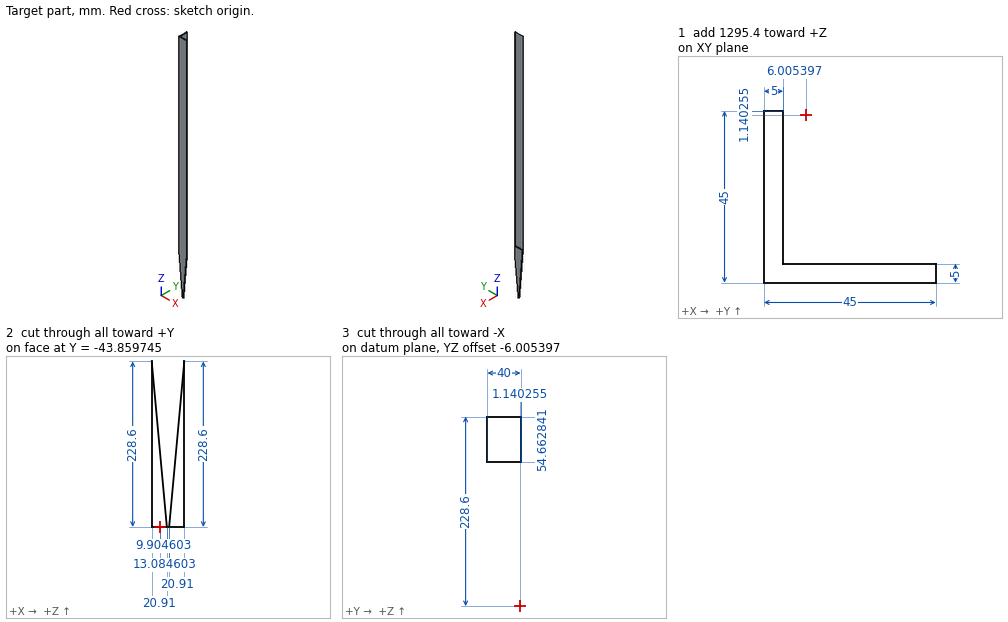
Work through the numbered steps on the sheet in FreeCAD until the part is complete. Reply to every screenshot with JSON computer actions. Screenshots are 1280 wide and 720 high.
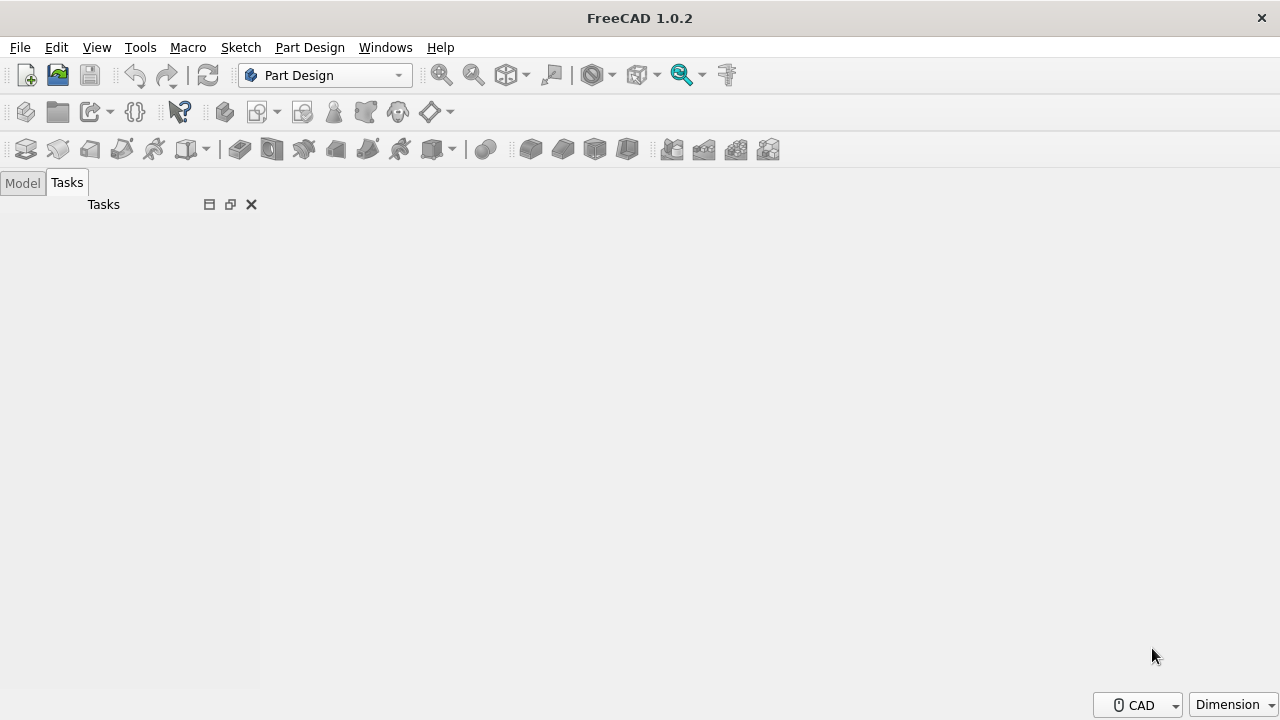
{"action": "key", "text": "ctrl+n"}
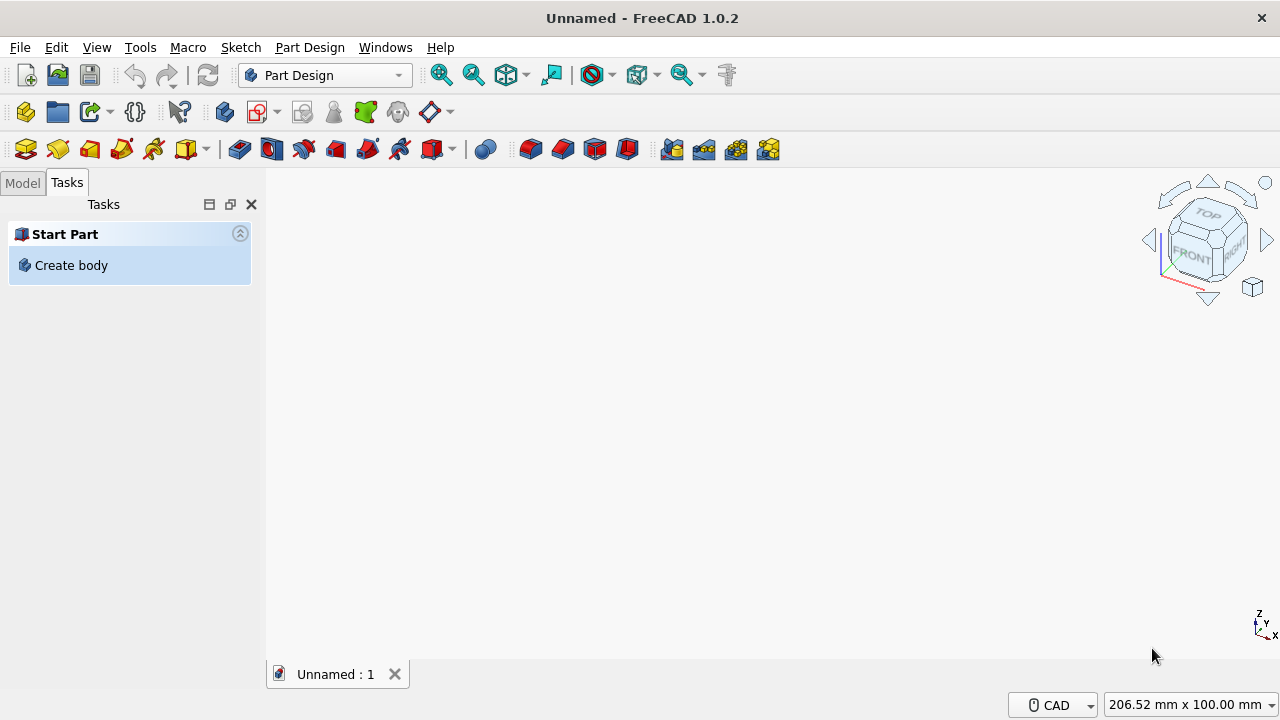
{"action": "left_click", "coordinate": [258, 112]}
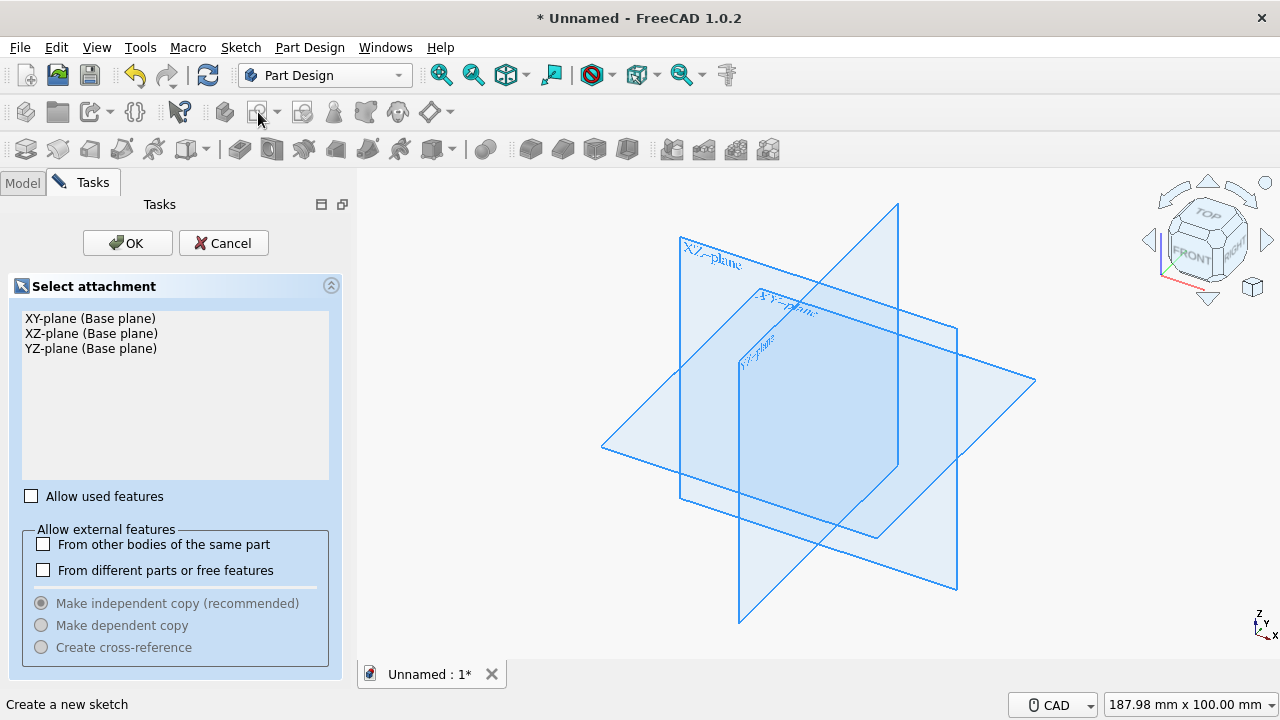
{"action": "left_click", "coordinate": [82, 318]}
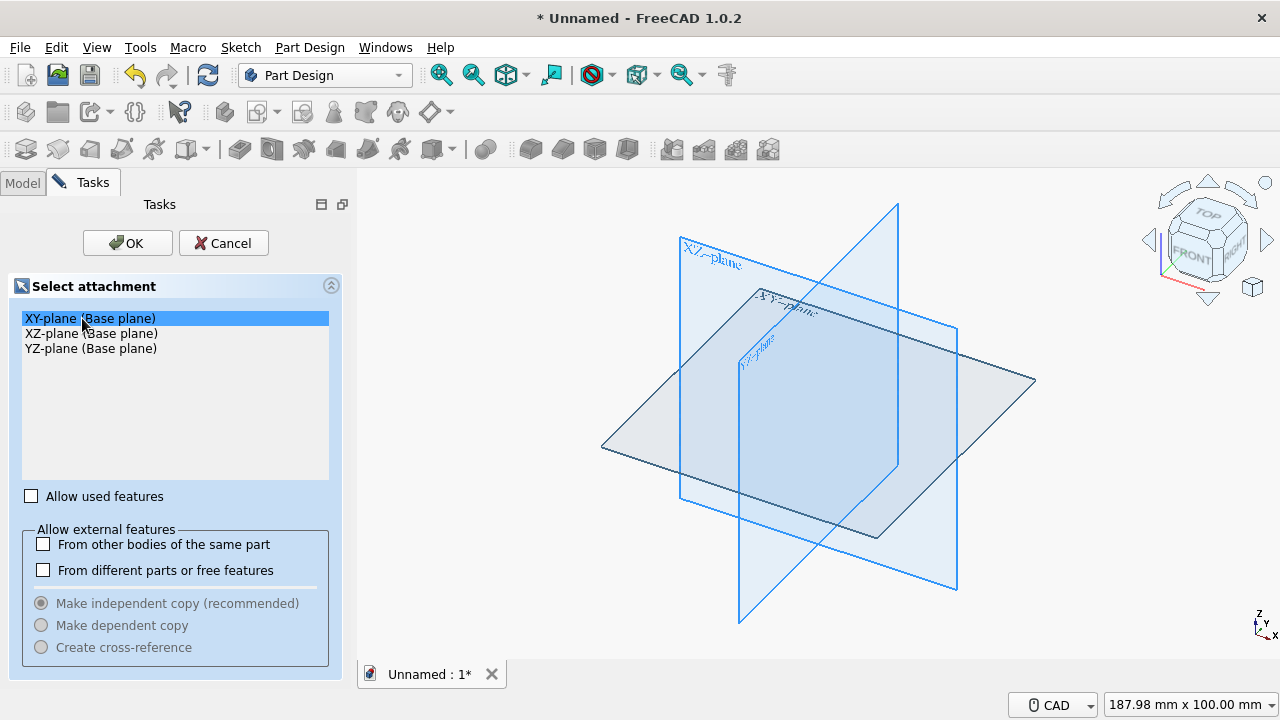
{"action": "left_click", "coordinate": [128, 243]}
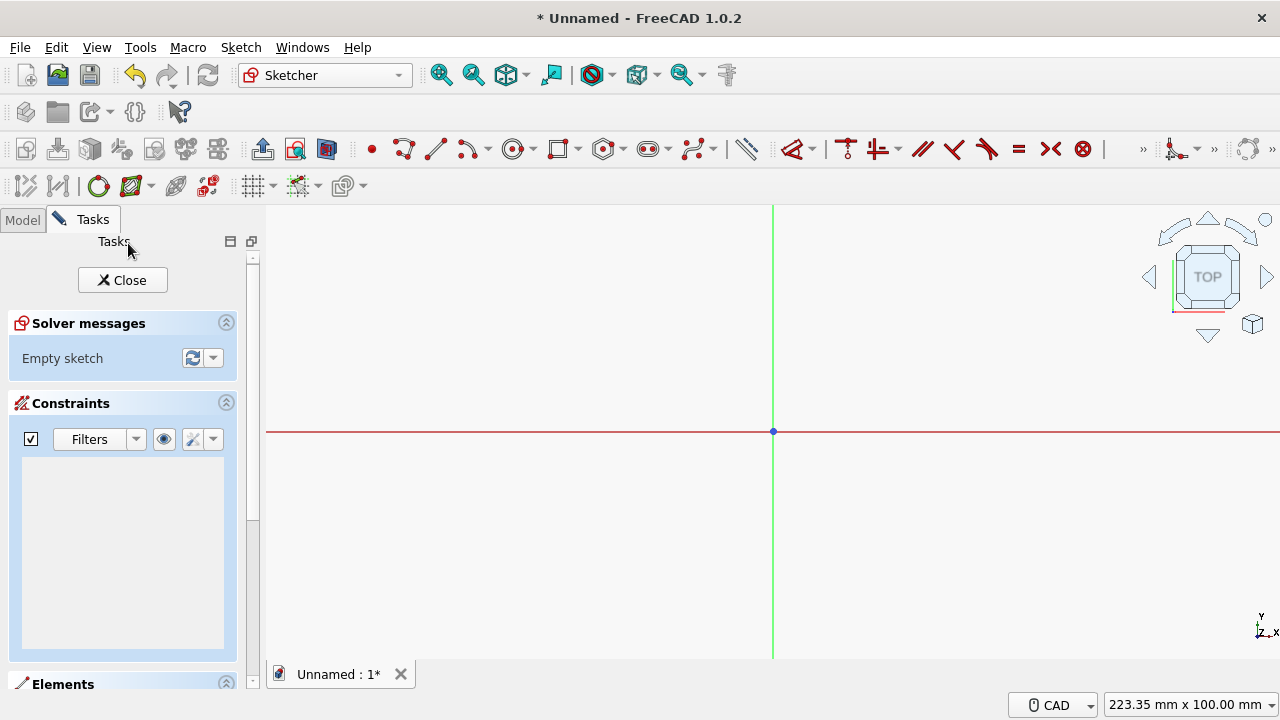
{"action": "scroll", "coordinate": [294, 233], "scroll_direction": "down", "scroll_amount": 1}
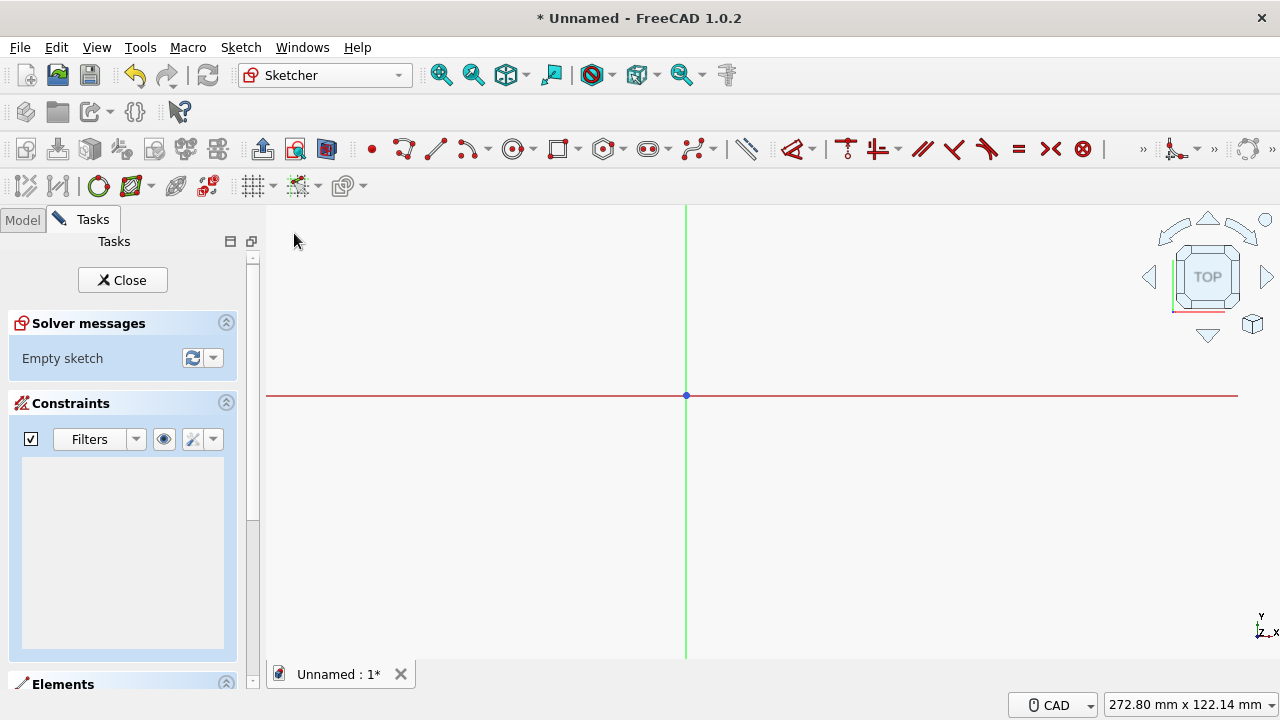
{"action": "scroll", "coordinate": [759, 528], "scroll_direction": "up", "scroll_amount": 3}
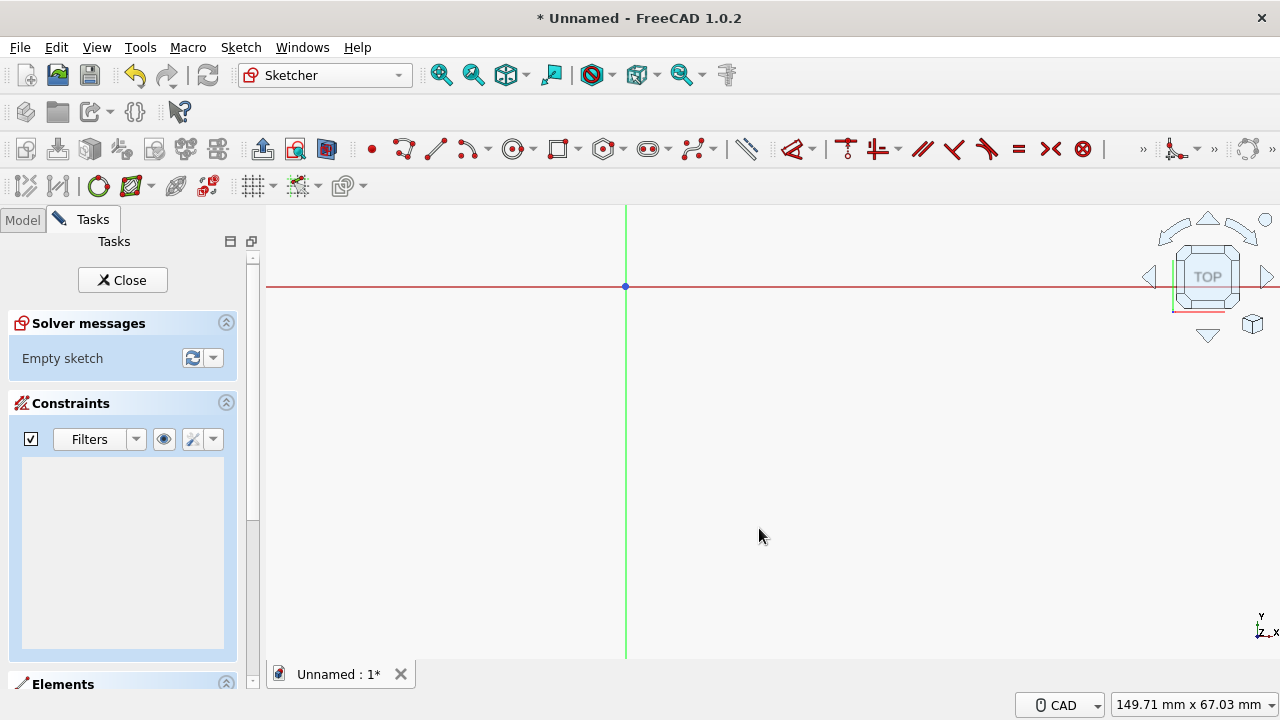
{"action": "key", "text": "g m"}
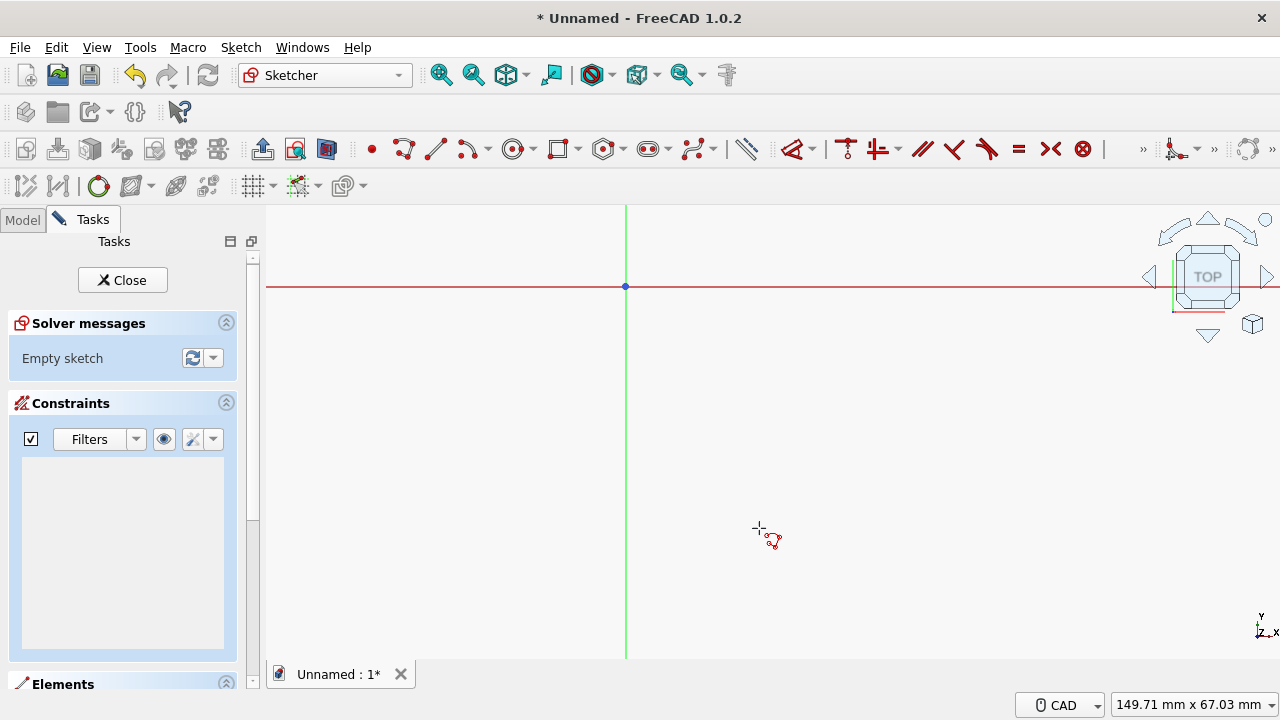
{"action": "scroll", "coordinate": [585, 279], "scroll_direction": "up", "scroll_amount": 4}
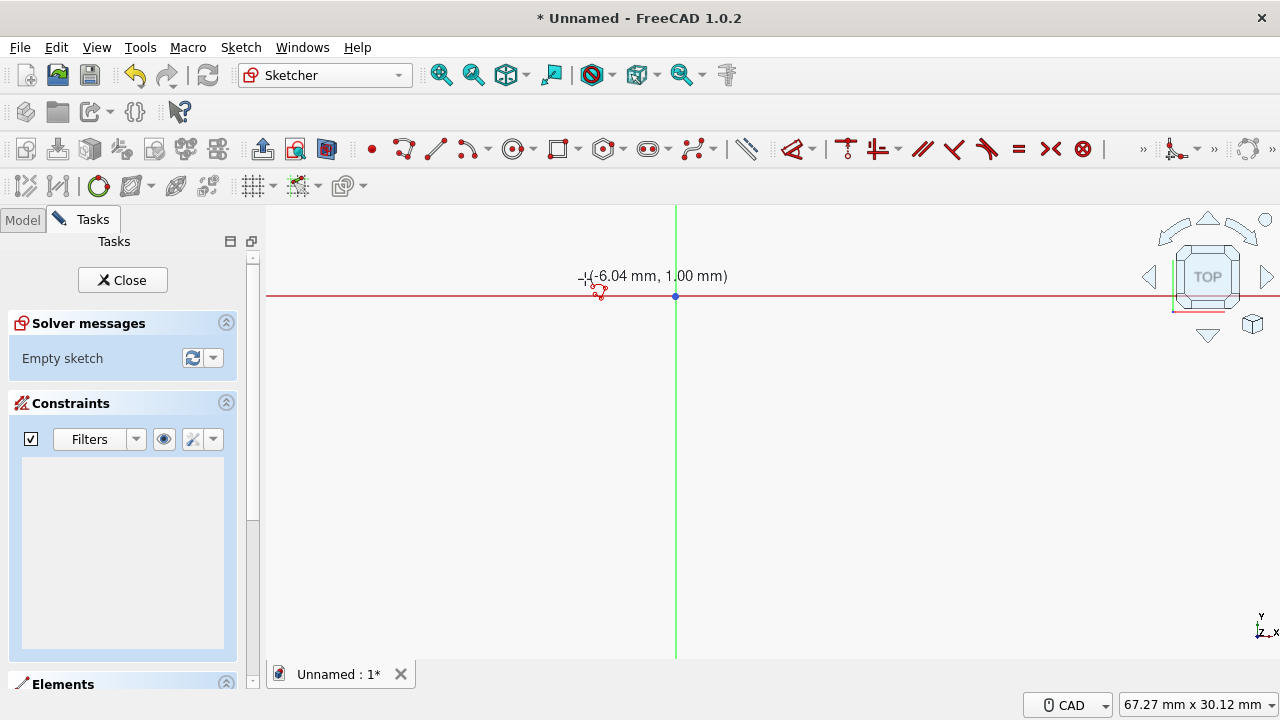
{"action": "left_click", "coordinate": [585, 279]}
{"action": "left_click", "coordinate": [510, 279]}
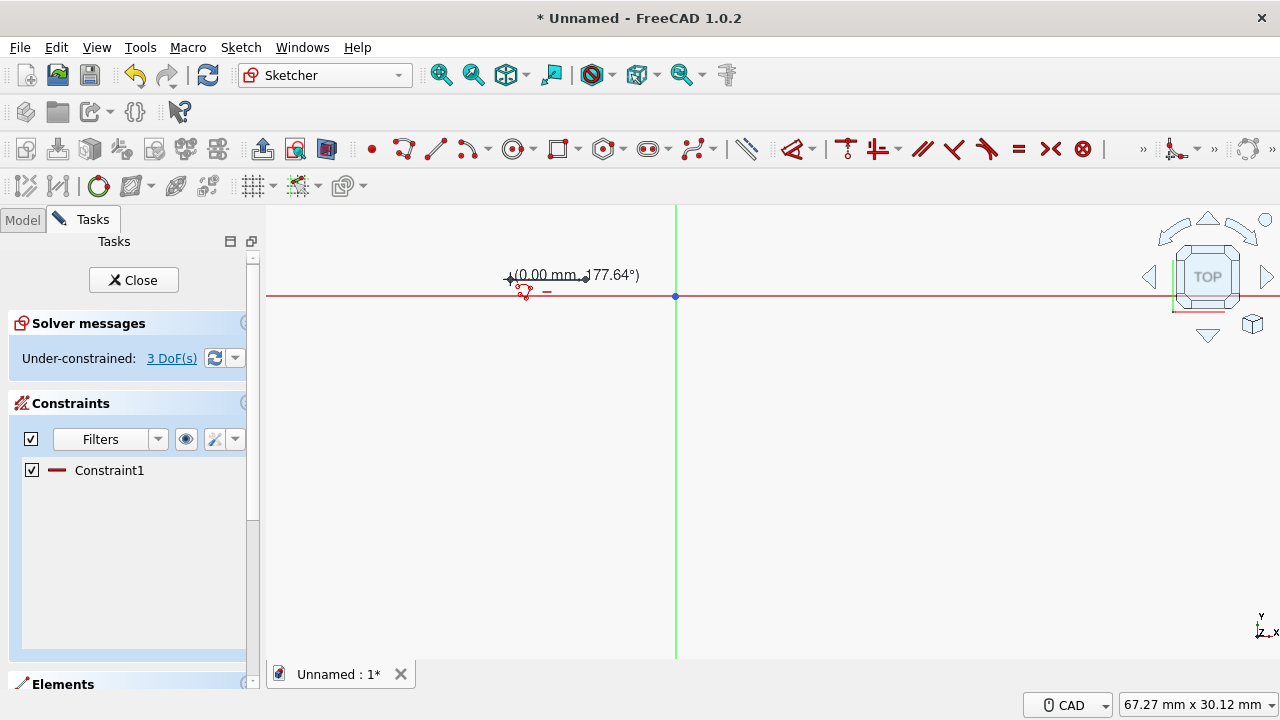
{"action": "scroll", "coordinate": [587, 280], "scroll_direction": "down", "scroll_amount": 4}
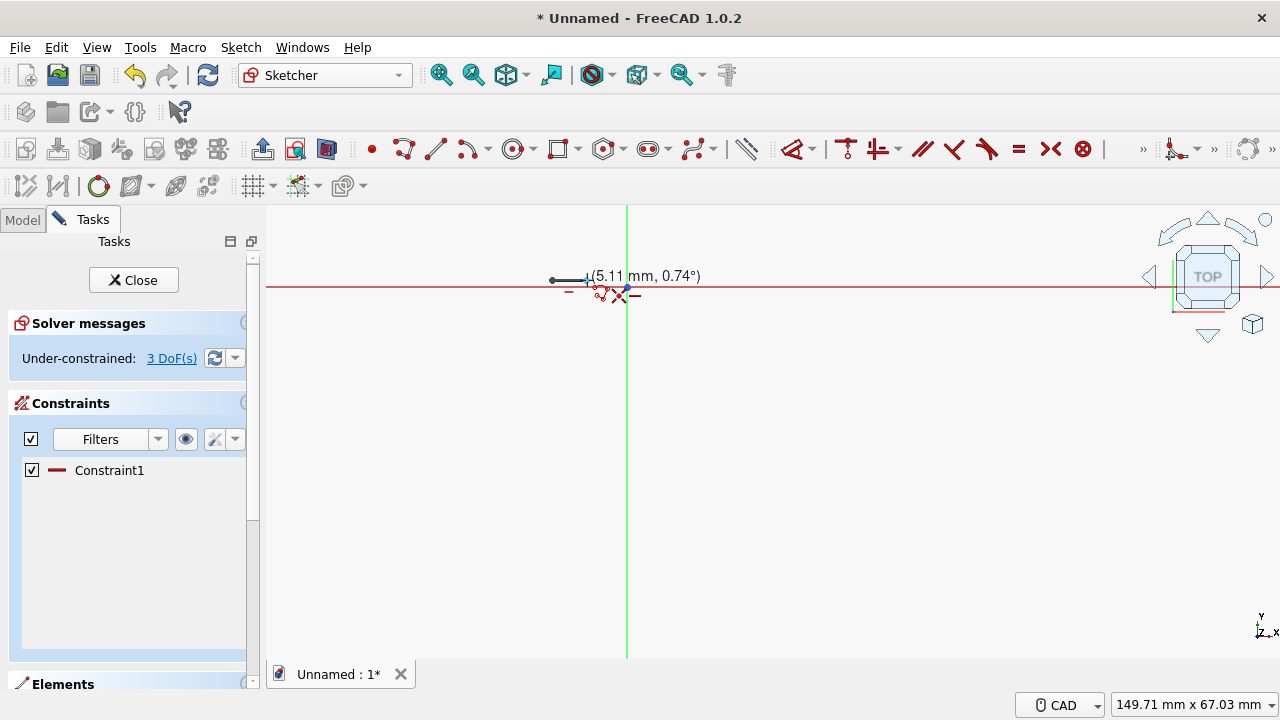
{"action": "left_click", "coordinate": [553, 584]}
{"action": "left_click", "coordinate": [857, 584]}
{"action": "left_click", "coordinate": [857, 551]}
{"action": "left_click", "coordinate": [586, 551]}